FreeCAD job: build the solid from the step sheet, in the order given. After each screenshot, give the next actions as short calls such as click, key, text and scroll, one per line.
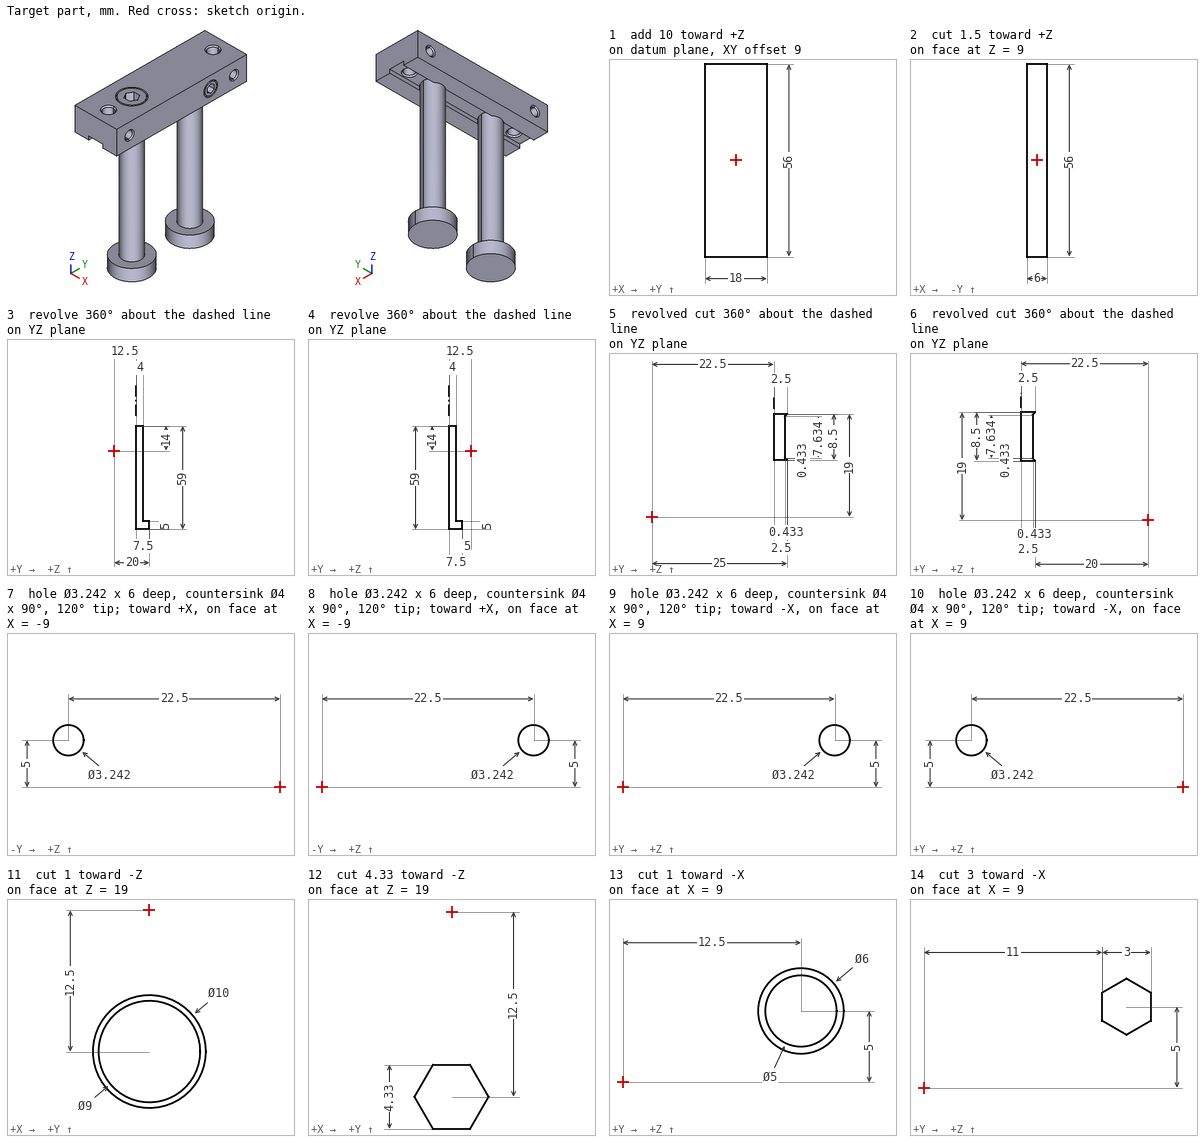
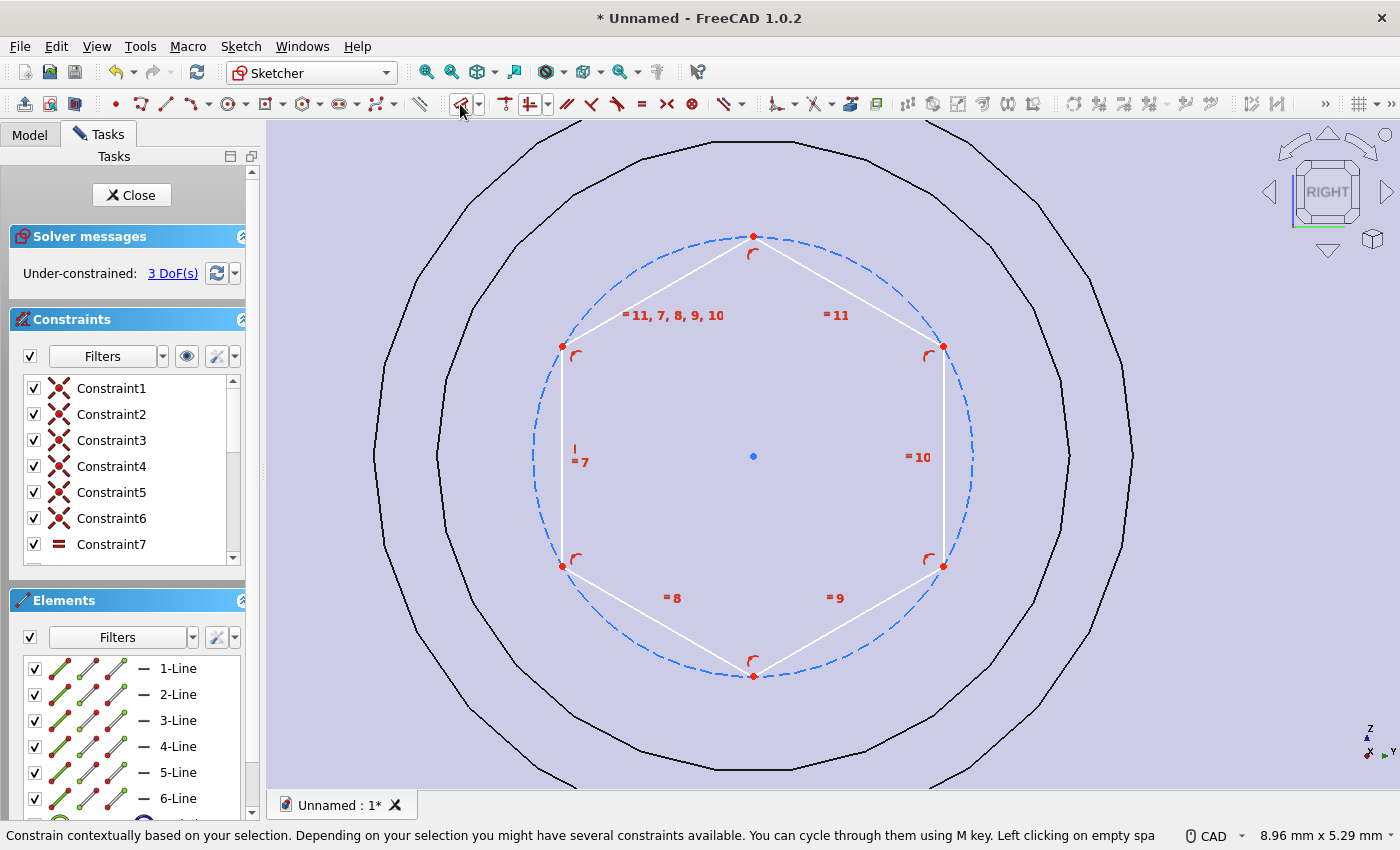
click(562, 347)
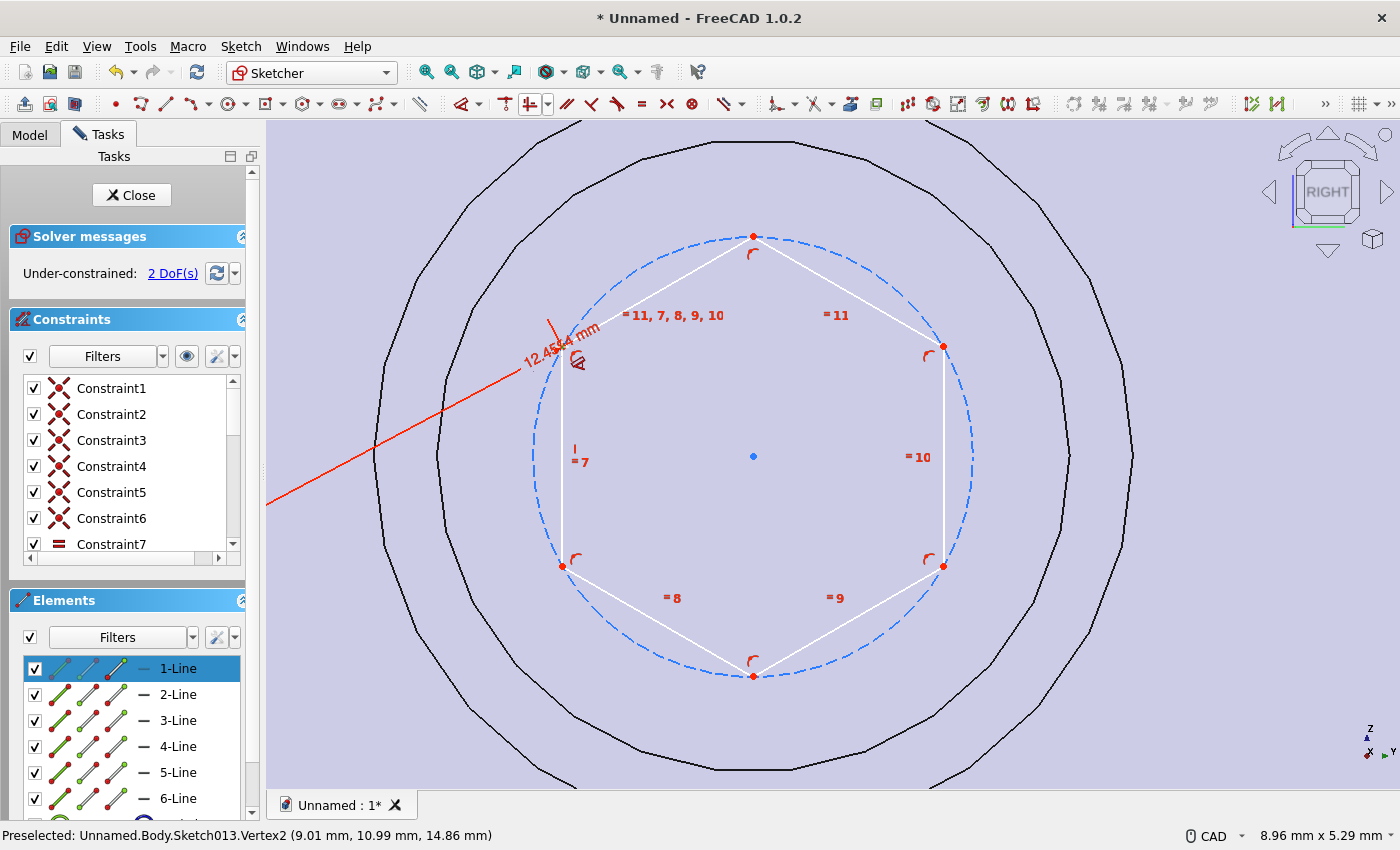
click(944, 567)
click(753, 601)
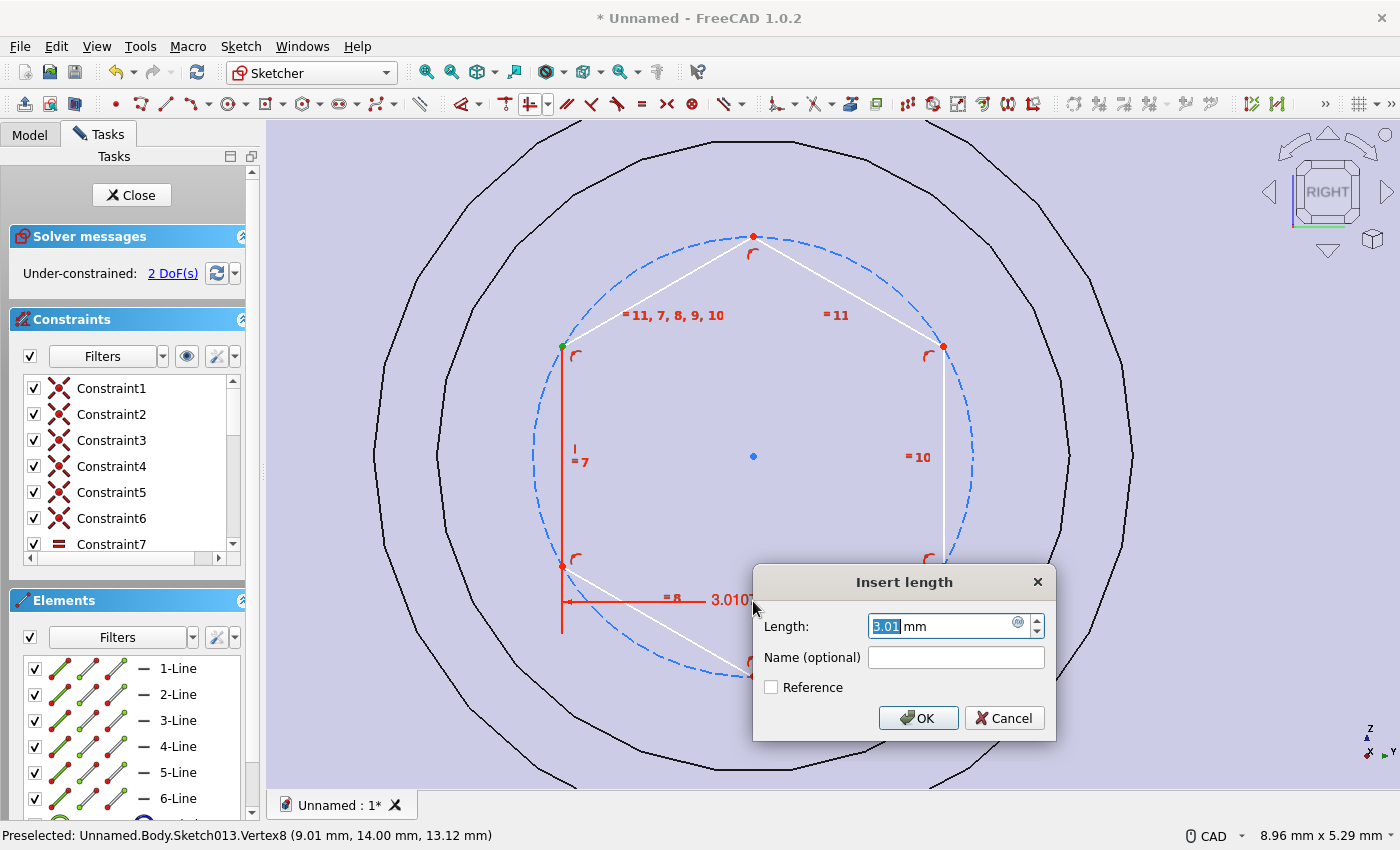
text(3)
key(Return)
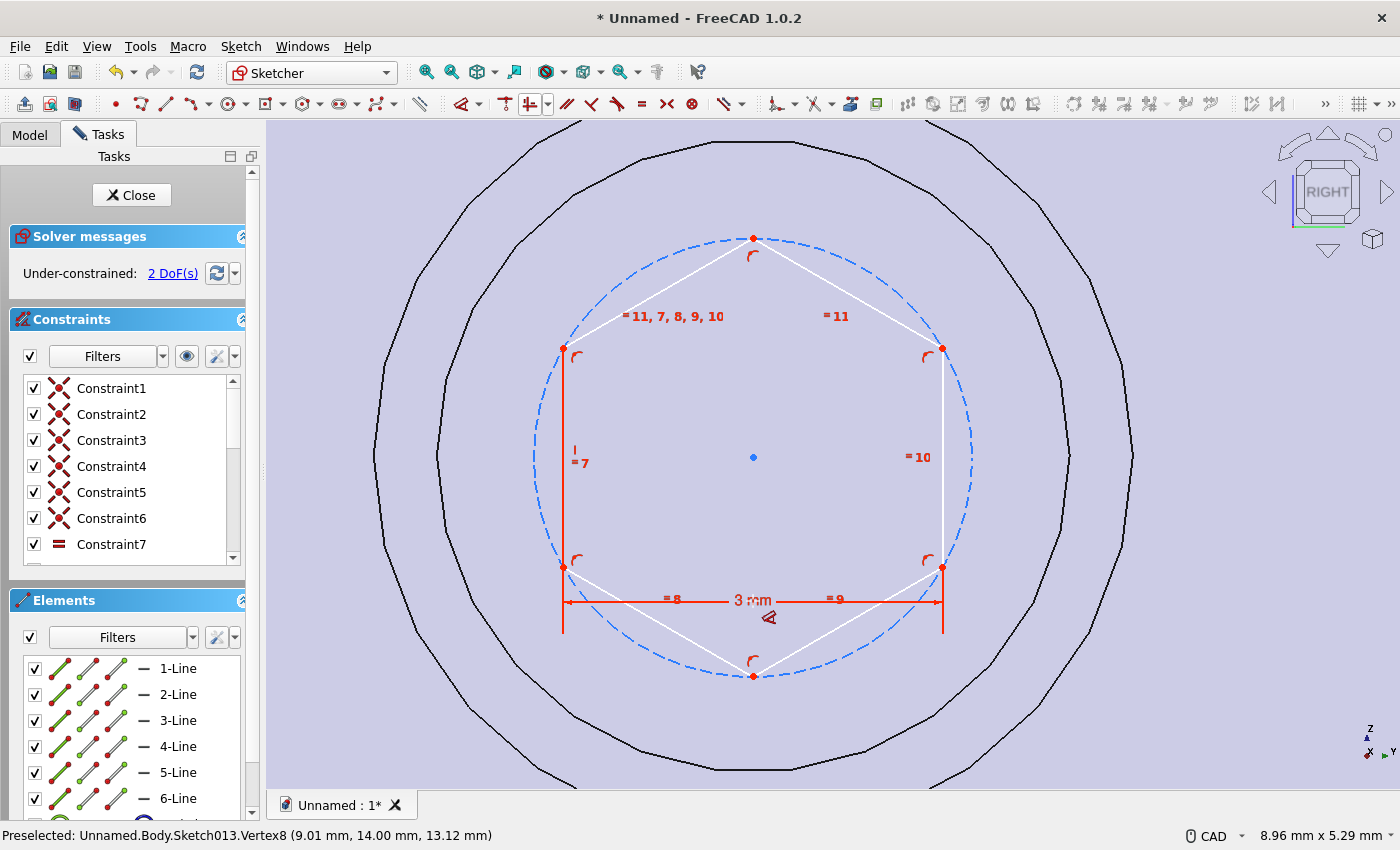
click(753, 458)
click(787, 540)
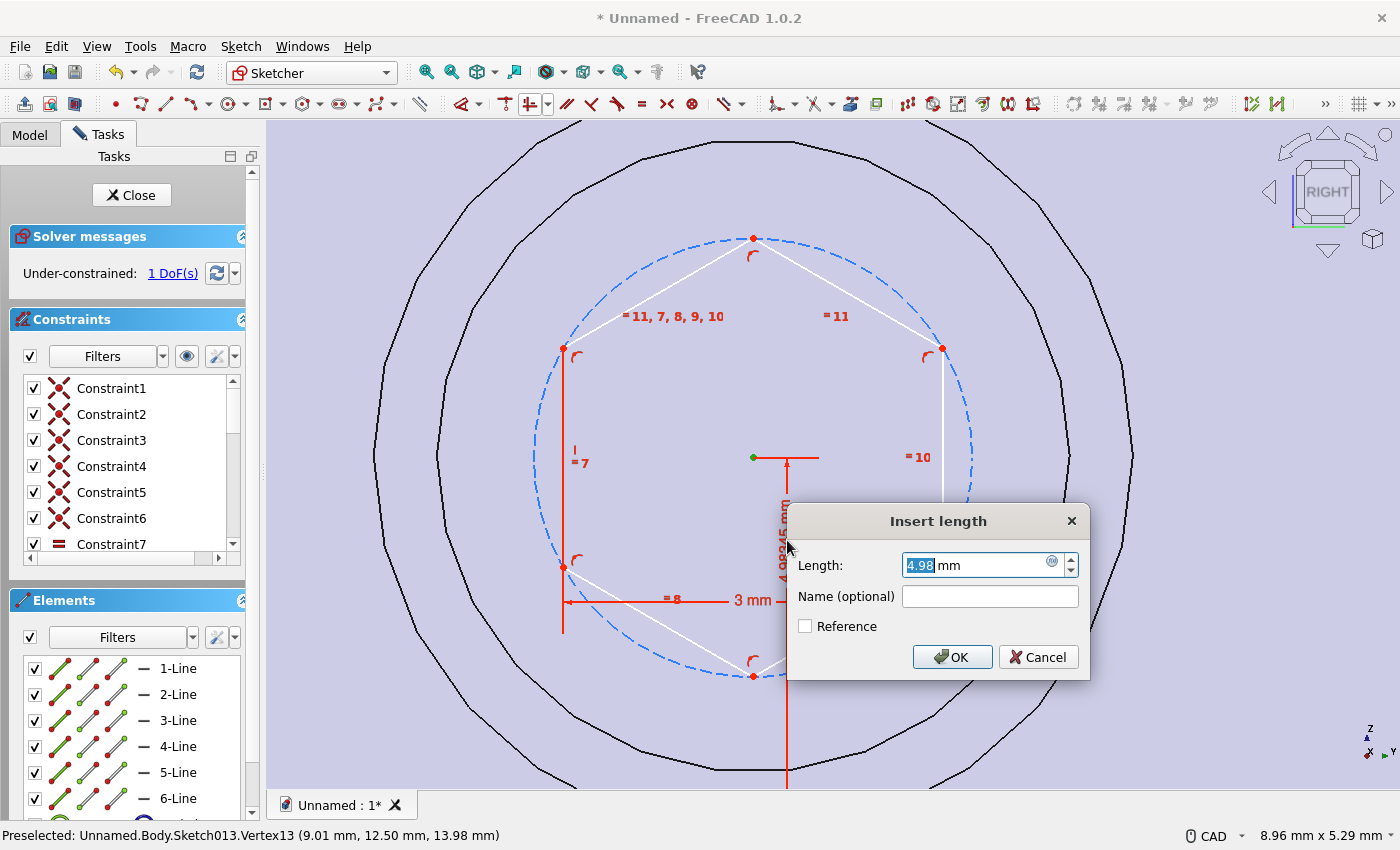
text(5)
key(Return)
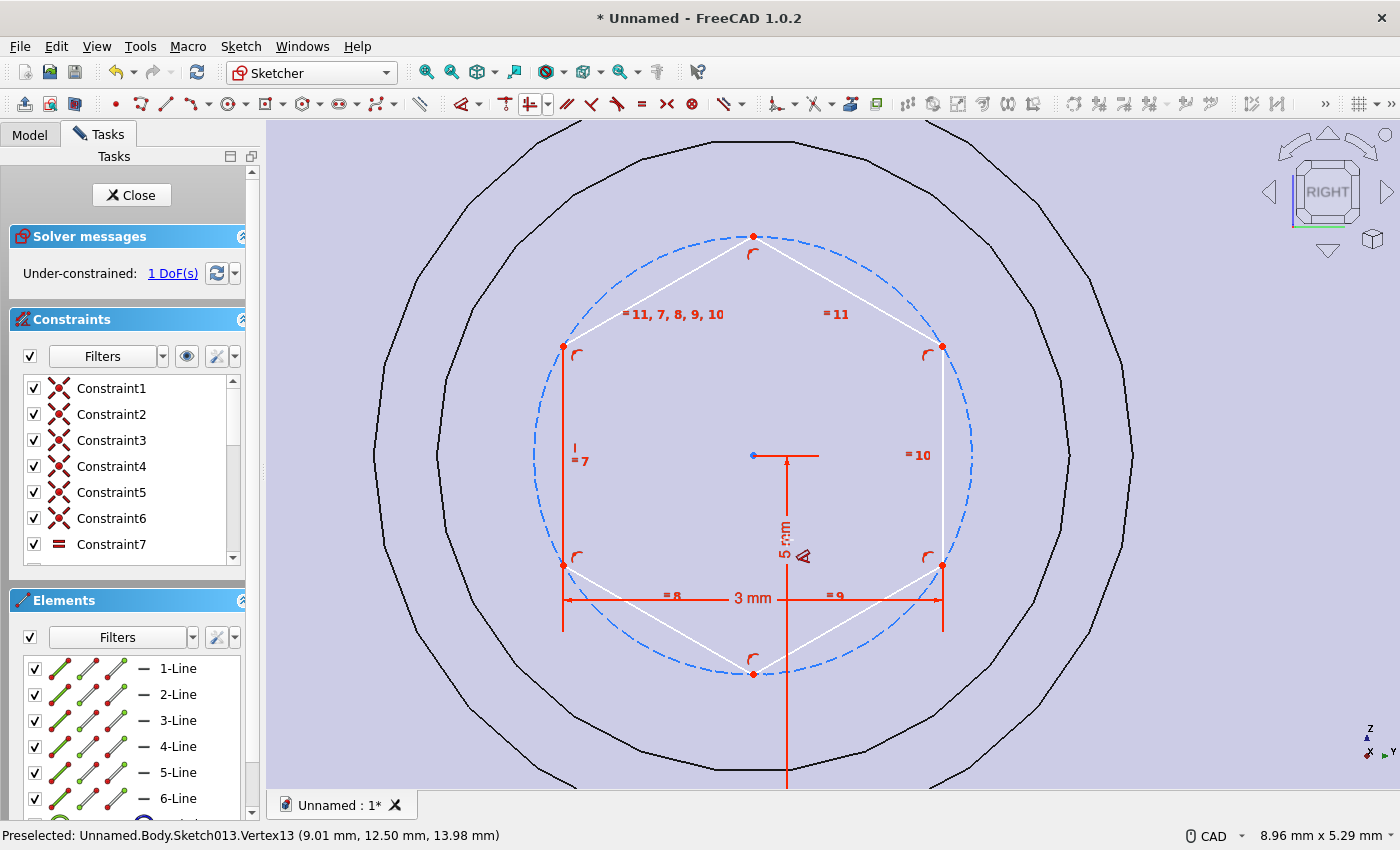
click(563, 346)
click(429, 312)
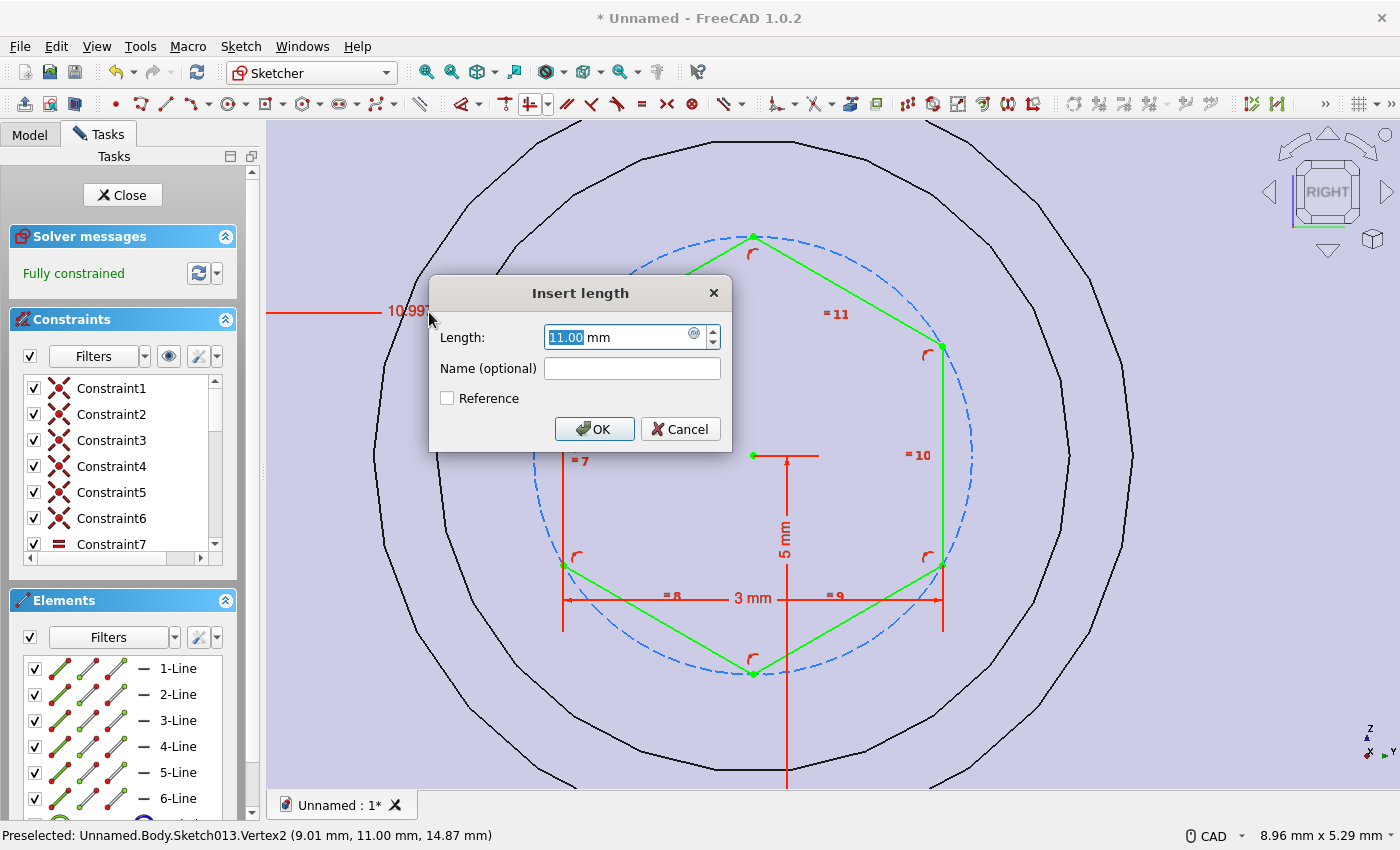
text(11)
key(Return)
key(Escape)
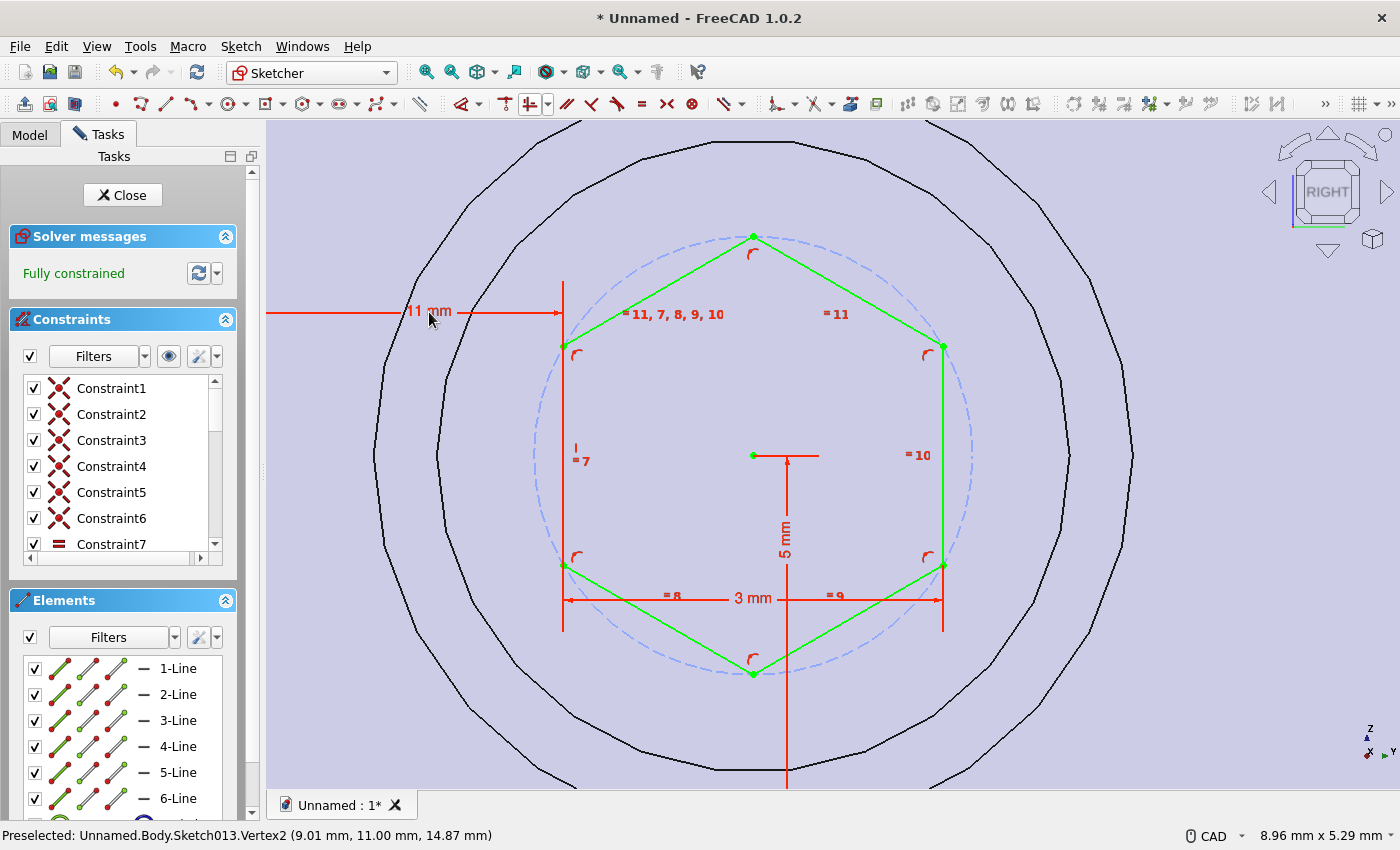
click(123, 195)